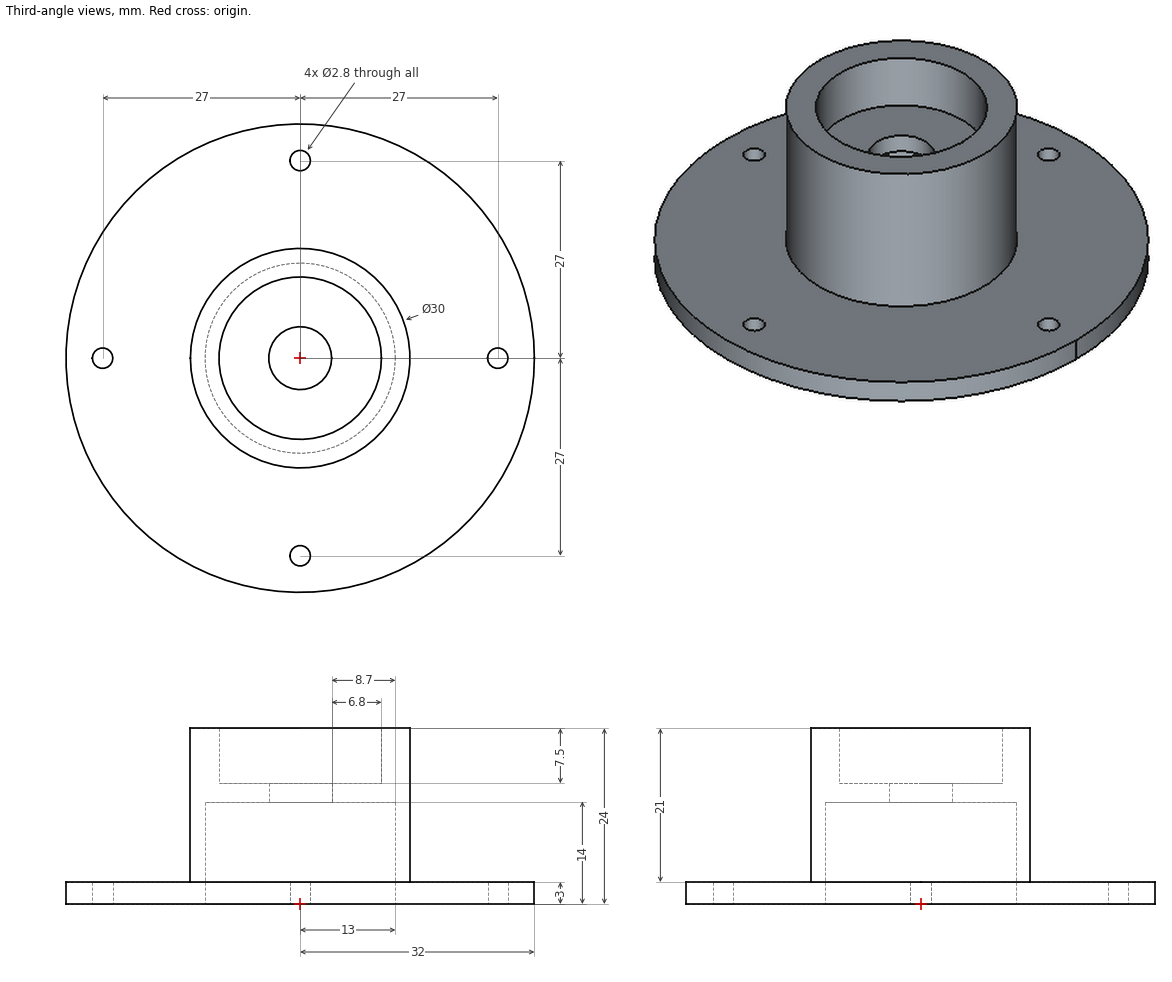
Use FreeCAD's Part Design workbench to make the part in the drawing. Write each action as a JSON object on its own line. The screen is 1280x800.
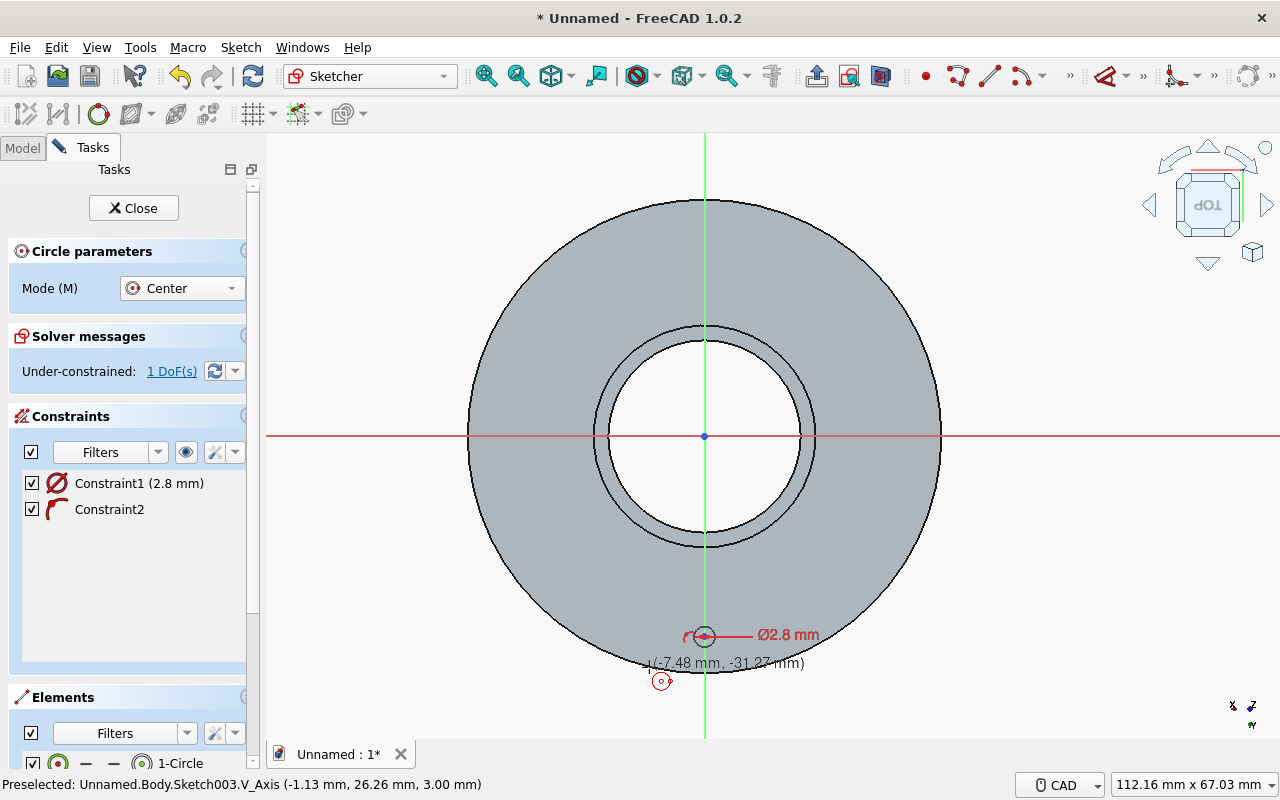
{"action": "scroll", "coordinate": [705, 237], "scroll_direction": "up", "scroll_amount": 4}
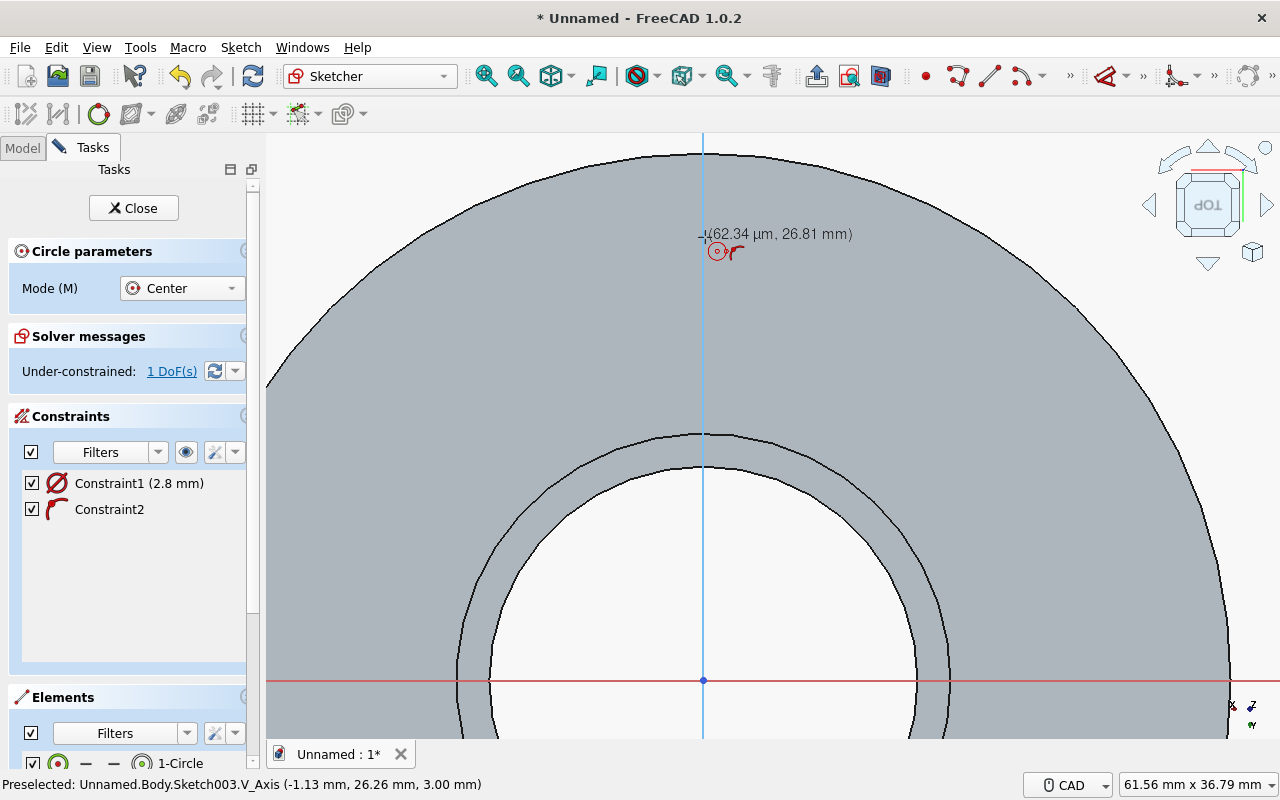
{"action": "left_click", "coordinate": [703, 236]}
{"action": "mouse_move", "coordinate": [720, 220]}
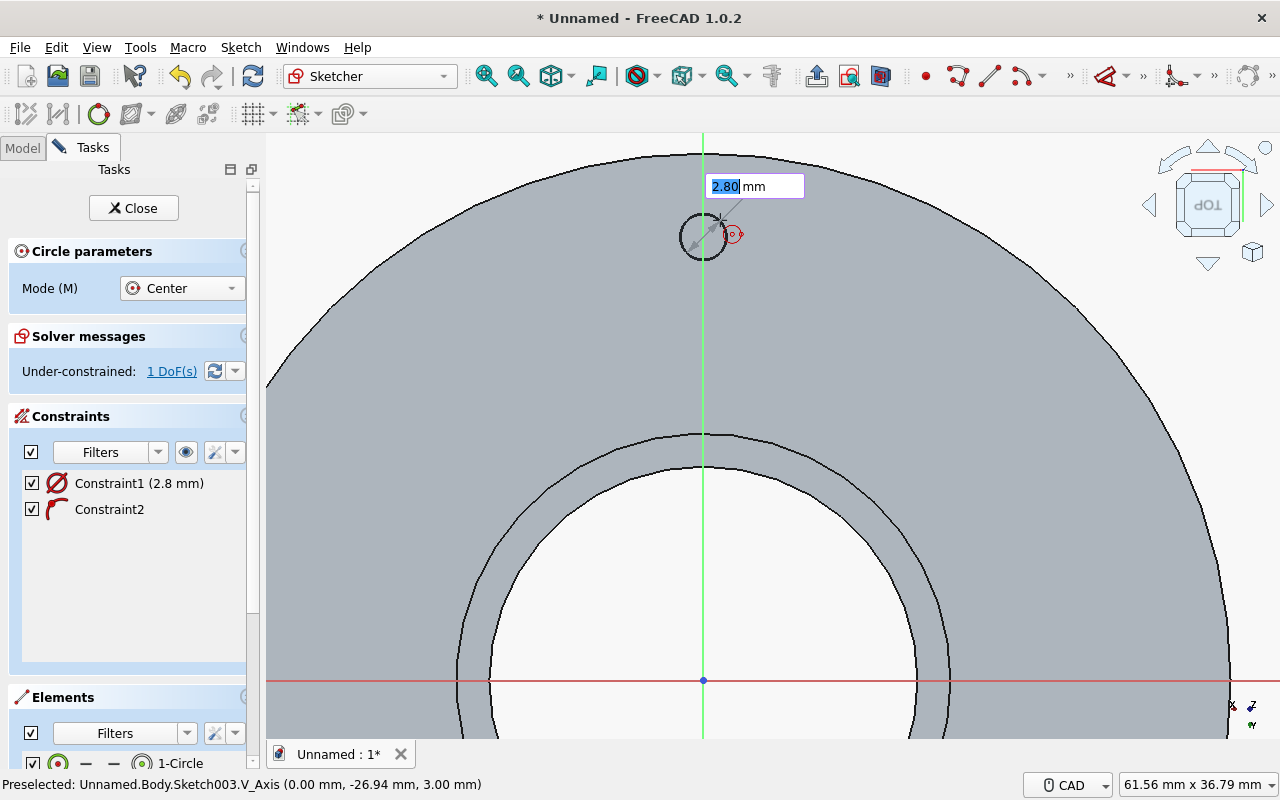
{"action": "type", "text": "2.8"}
{"action": "key", "text": "Return"}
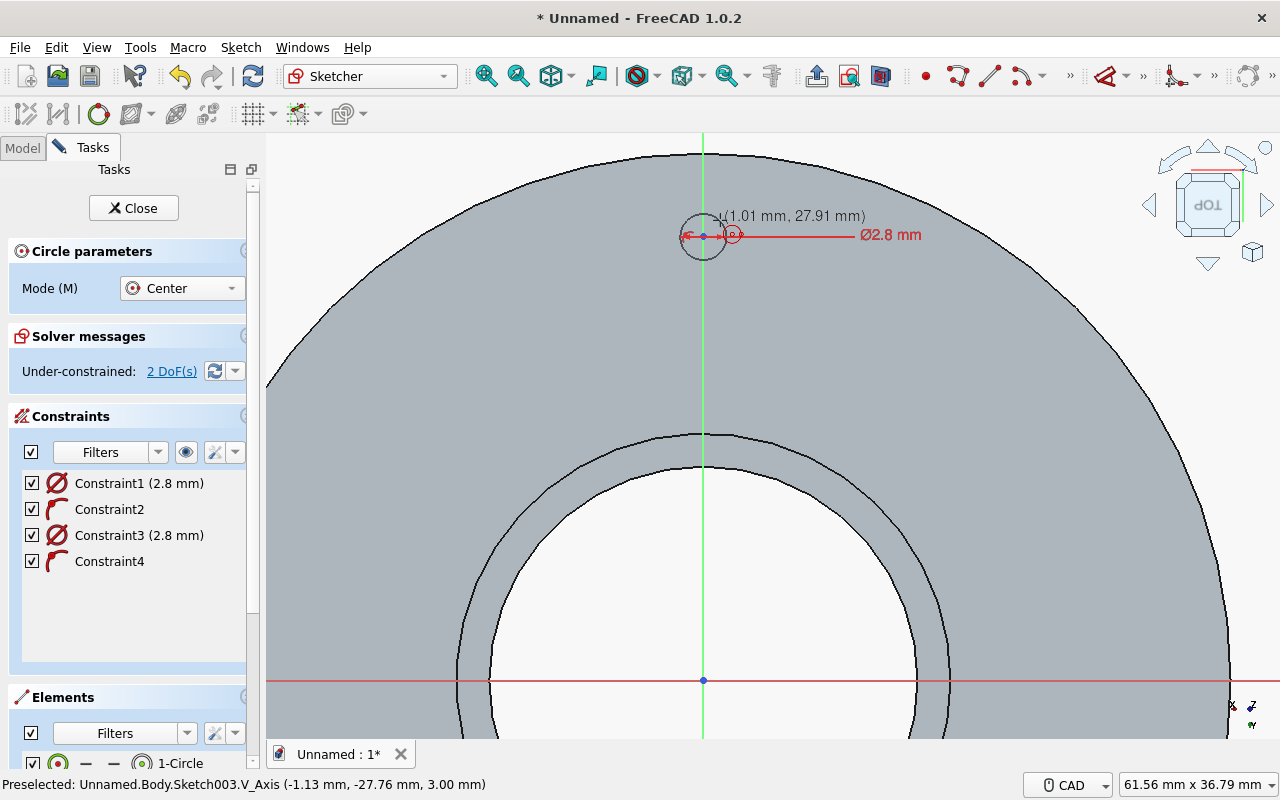
{"action": "scroll", "coordinate": [705, 236], "scroll_direction": "down", "scroll_amount": 4}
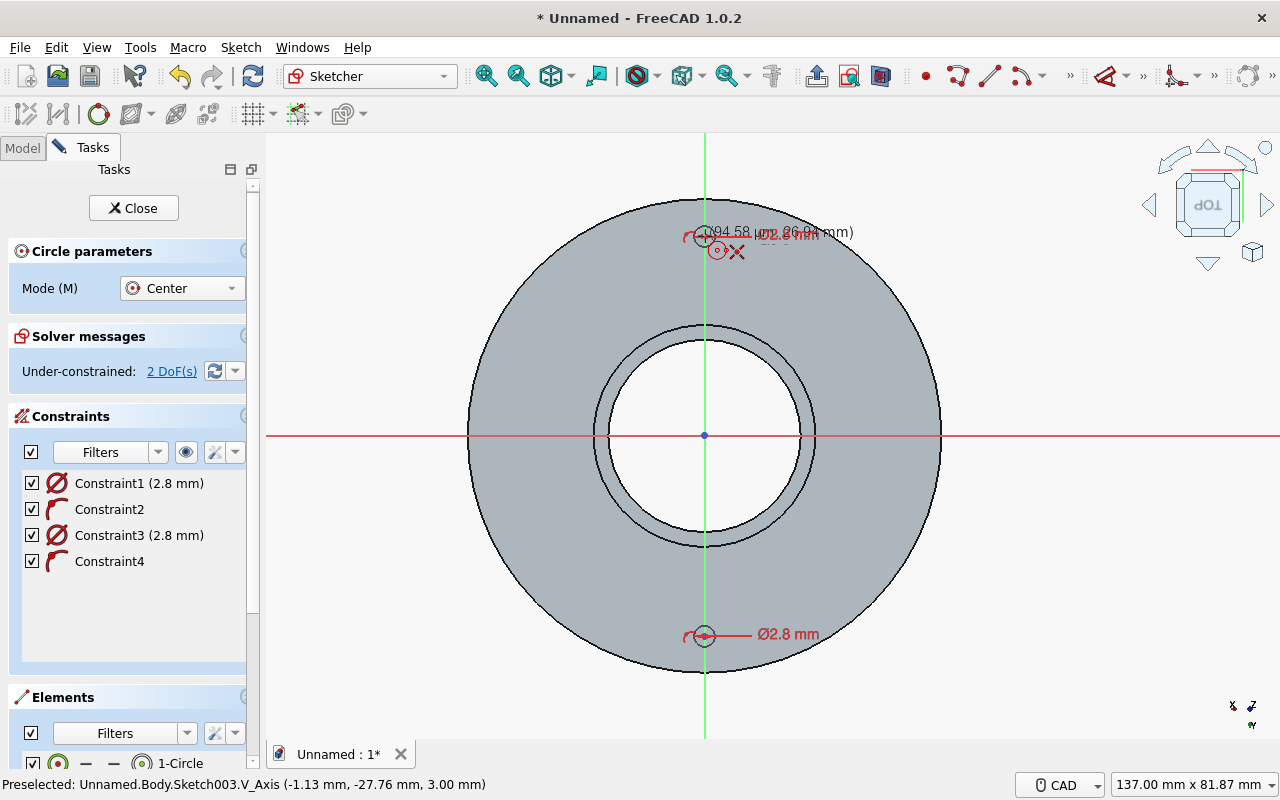
{"action": "scroll", "coordinate": [505, 436], "scroll_direction": "up", "scroll_amount": 4}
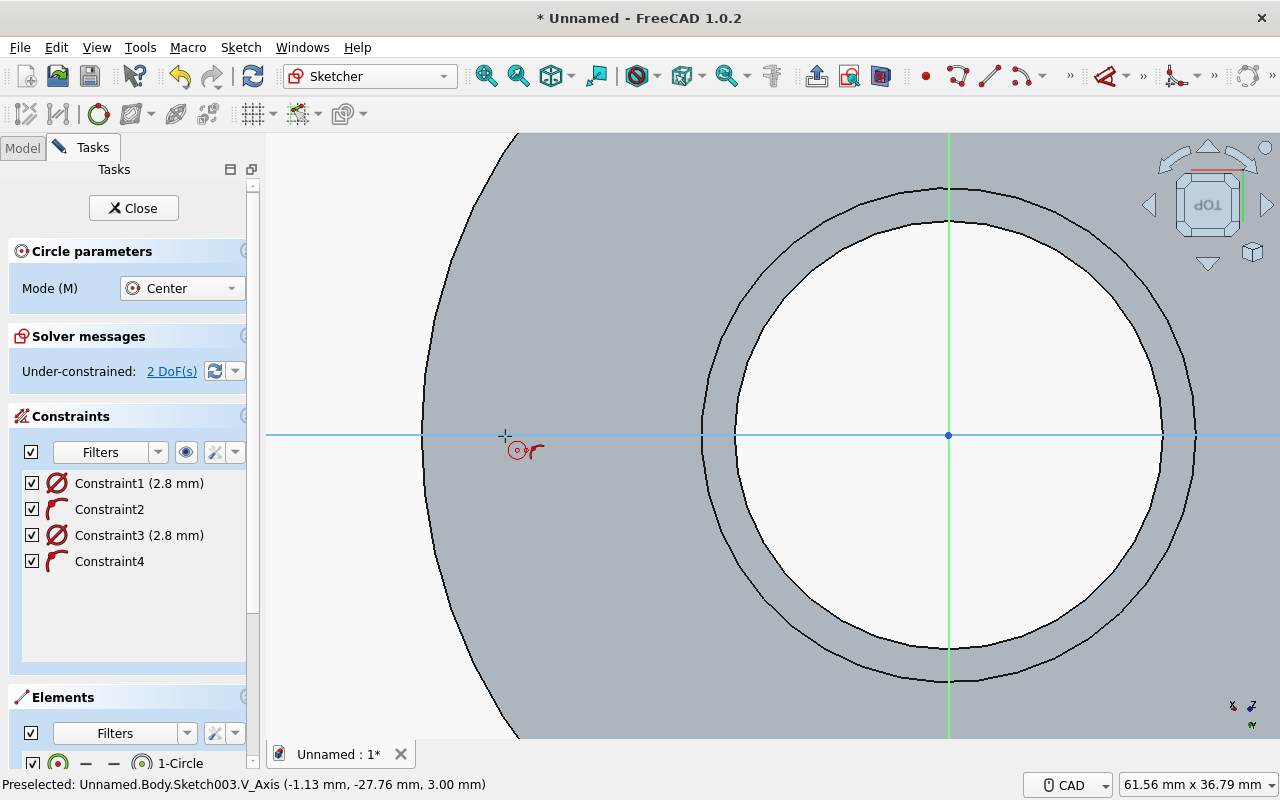
{"action": "left_click", "coordinate": [504, 435]}
{"action": "mouse_move", "coordinate": [520, 419]}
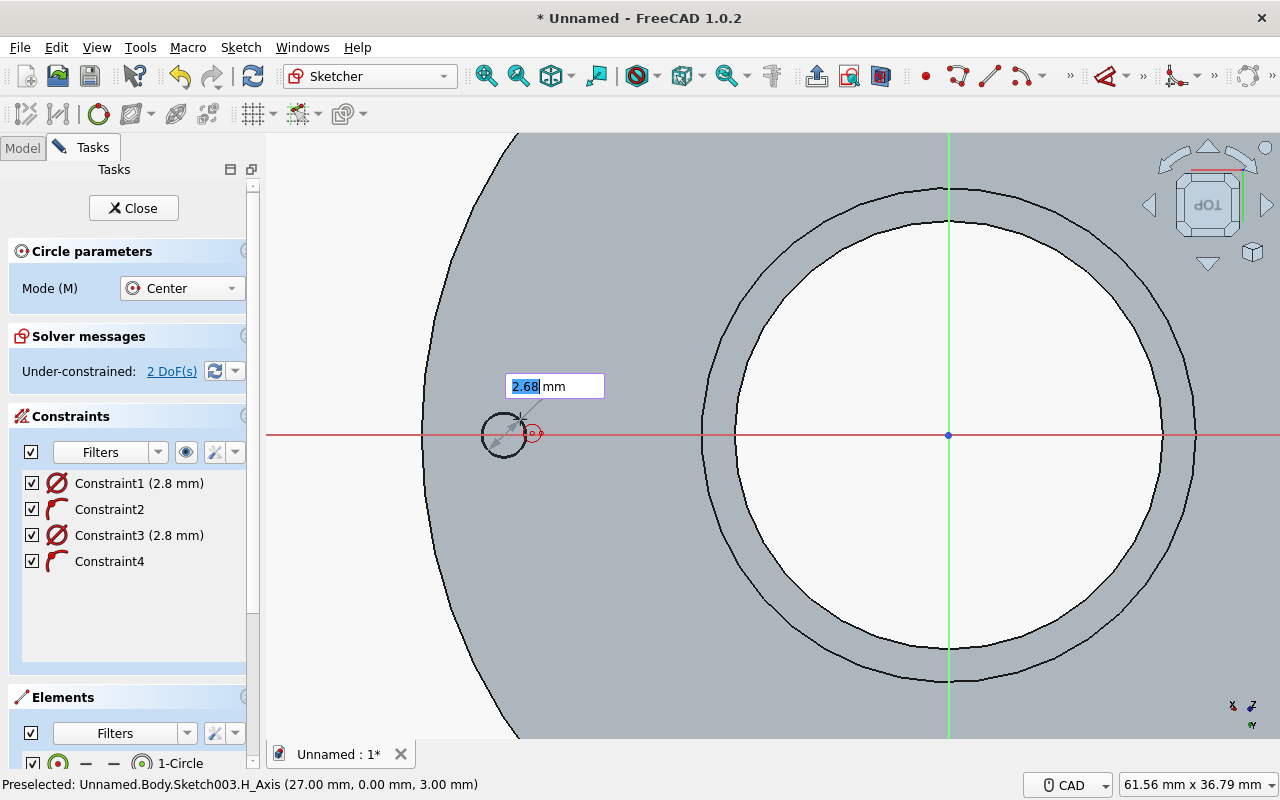
{"action": "type", "text": "2.8"}
{"action": "key", "text": "Return"}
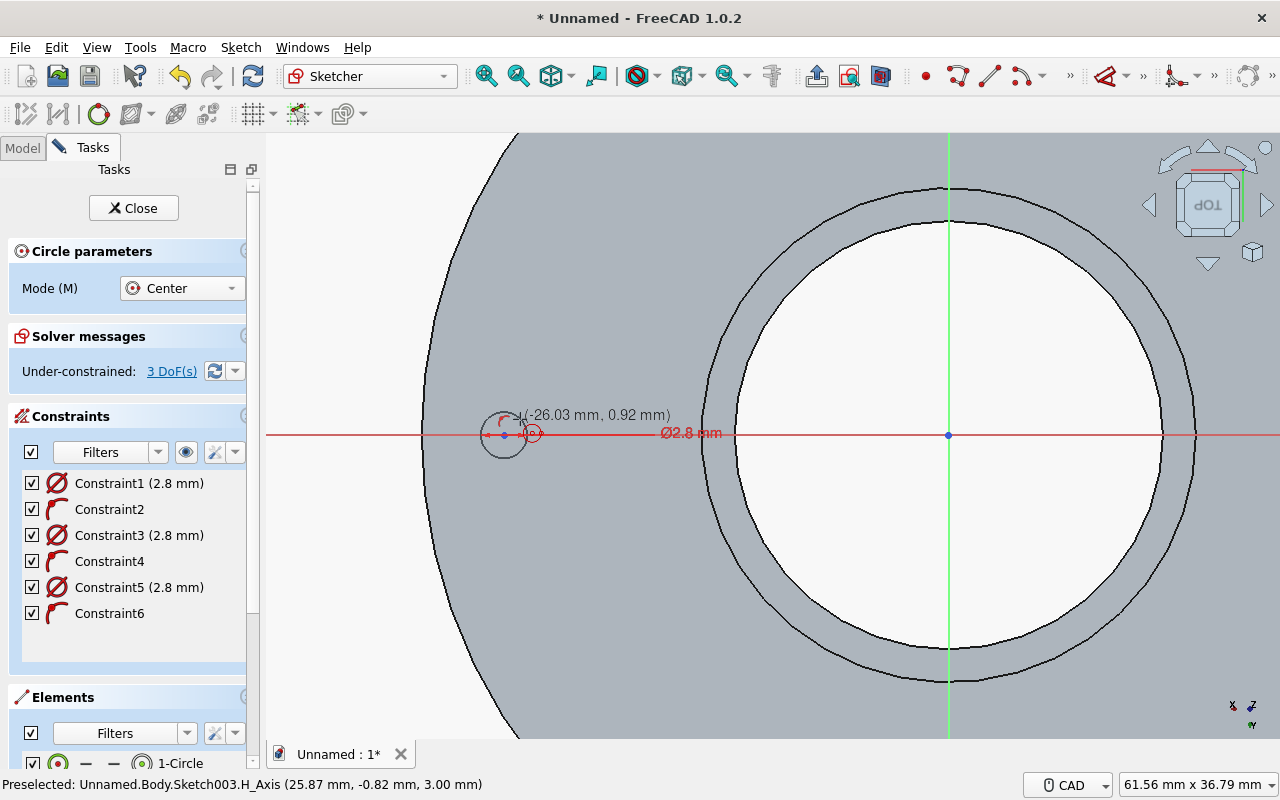
{"action": "scroll", "coordinate": [505, 437], "scroll_direction": "down", "scroll_amount": 4}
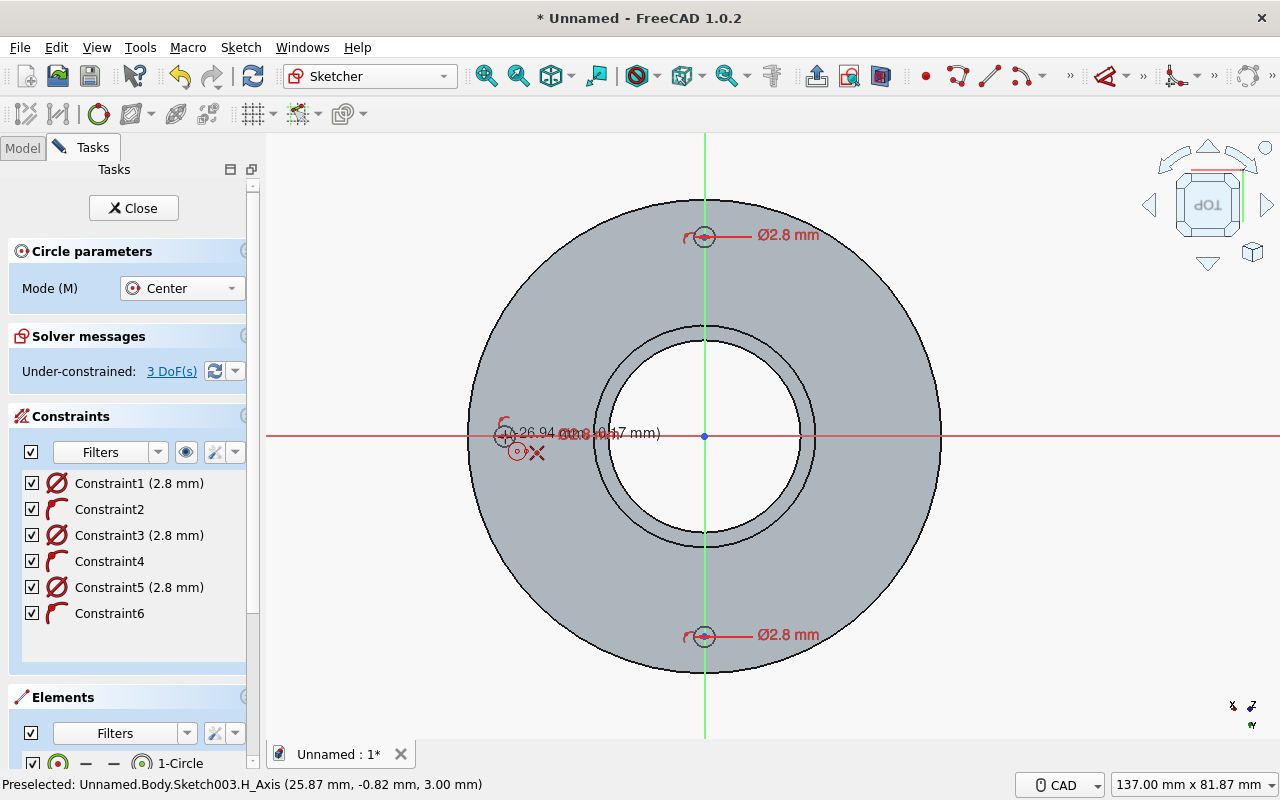
{"action": "scroll", "coordinate": [904, 436], "scroll_direction": "up", "scroll_amount": 4}